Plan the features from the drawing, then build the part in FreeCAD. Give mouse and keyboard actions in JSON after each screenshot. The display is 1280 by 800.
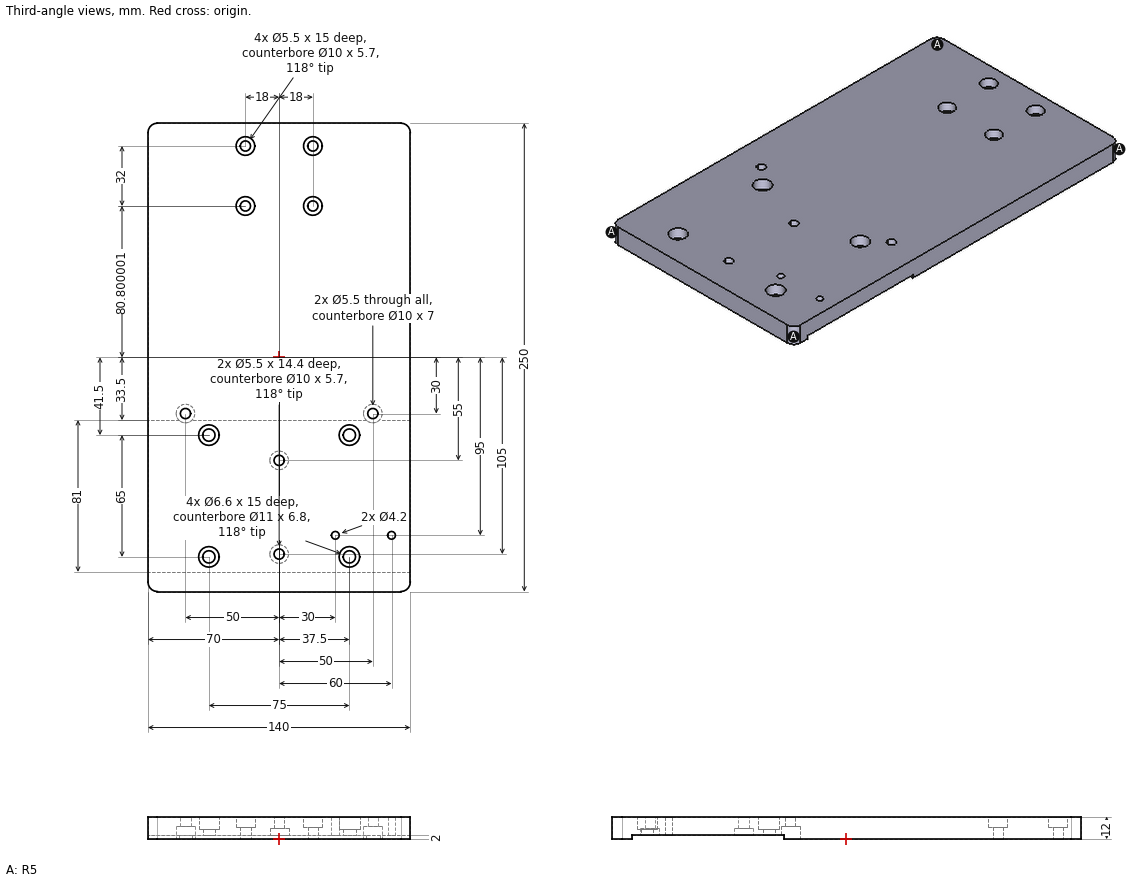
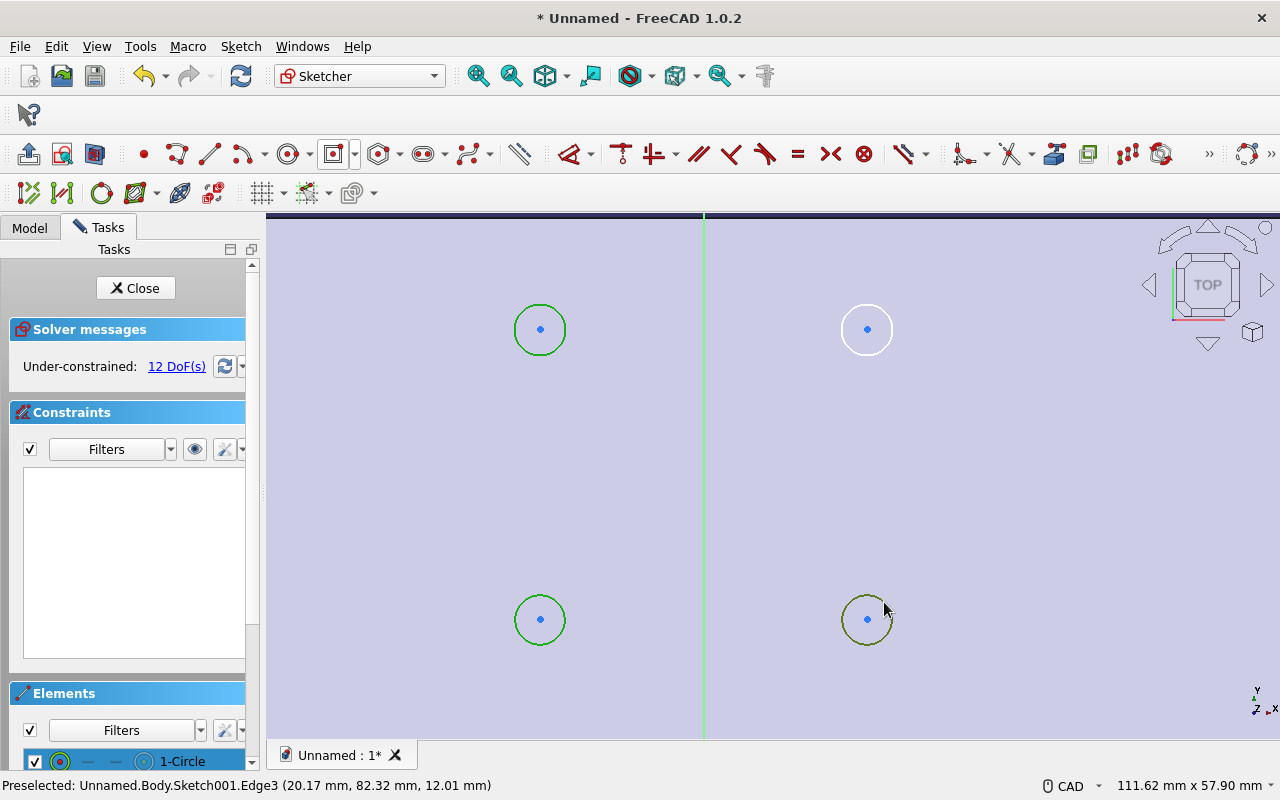
{"action": "left_click", "coordinate": [885, 312]}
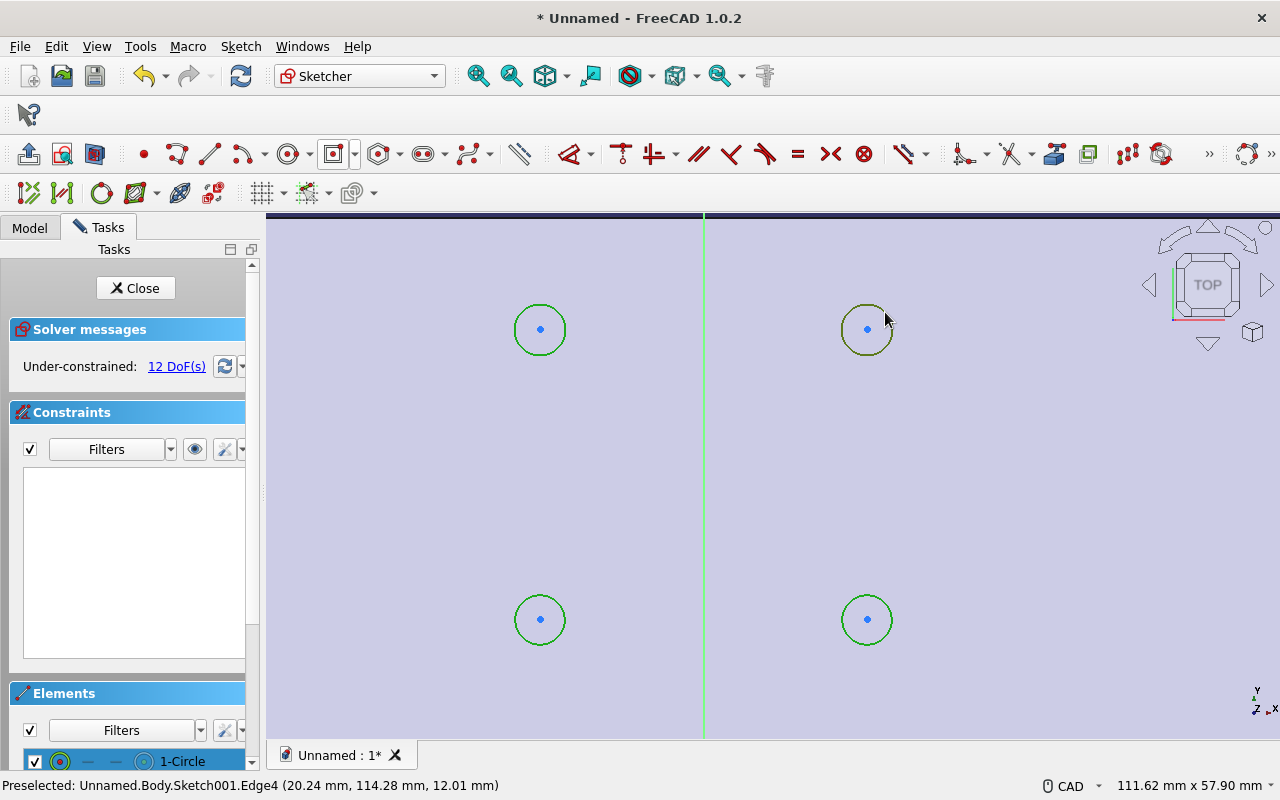
{"action": "left_click", "coordinate": [798, 154]}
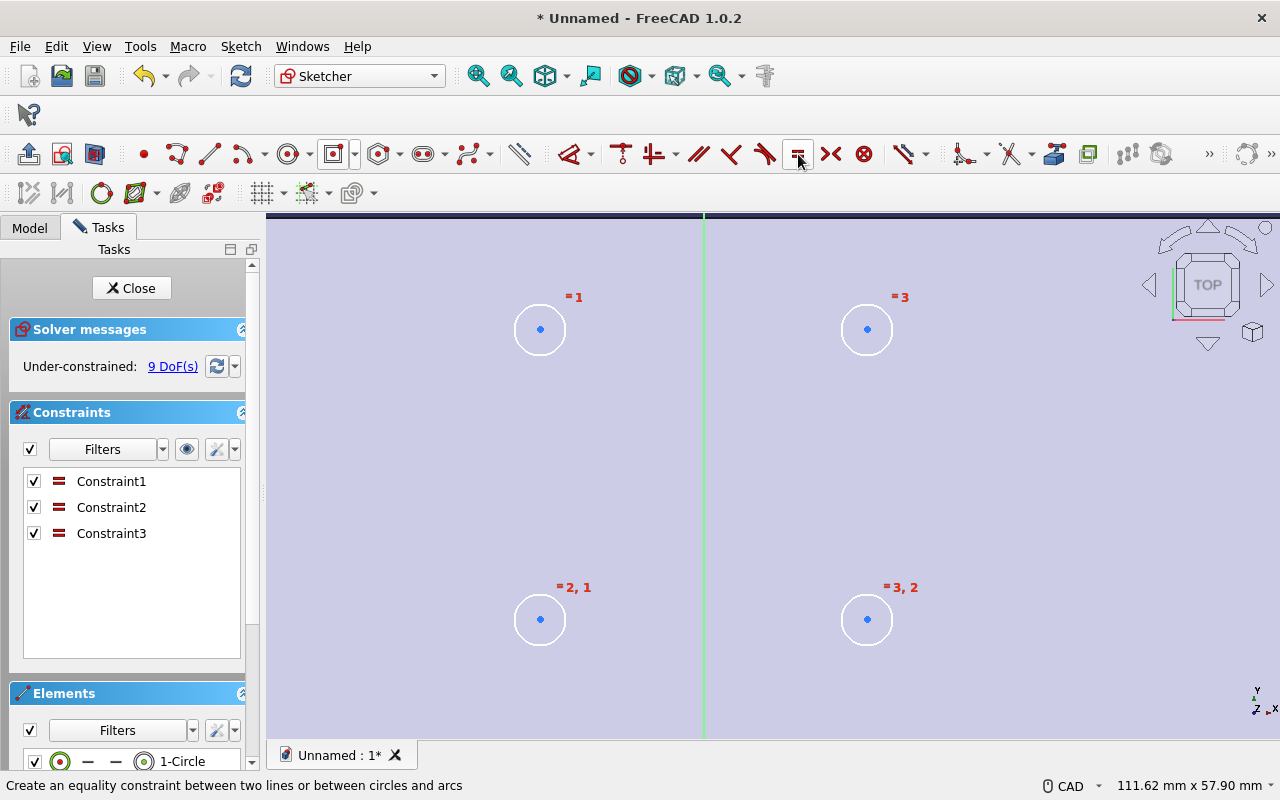
{"action": "left_click", "coordinate": [540, 330]}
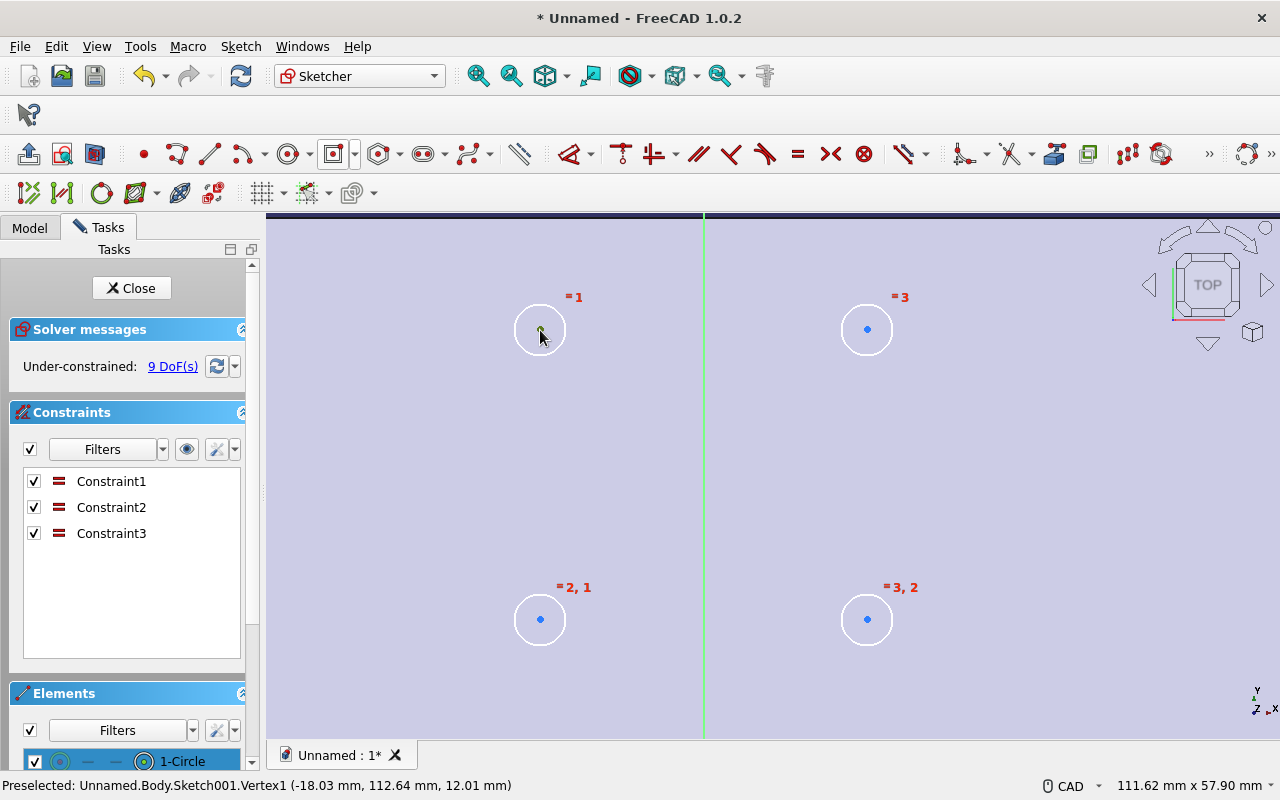
{"action": "left_click", "coordinate": [540, 620]}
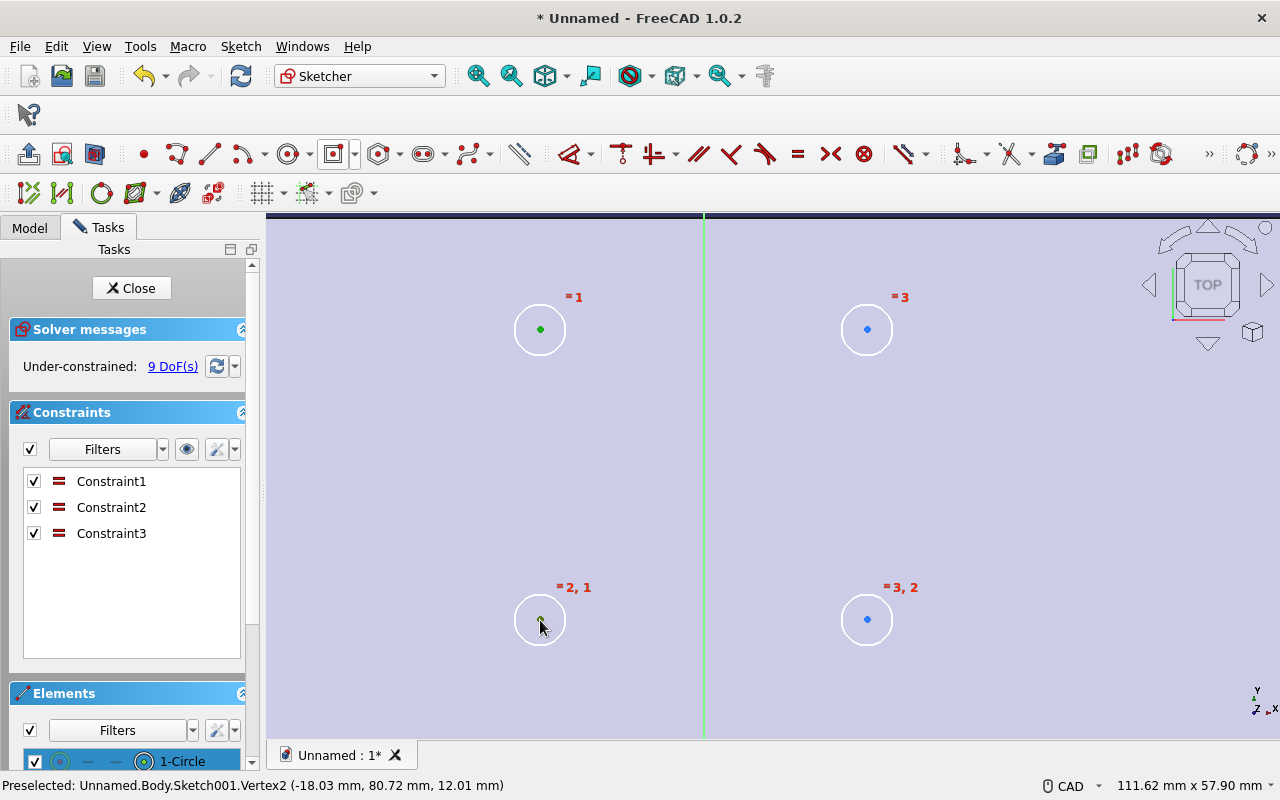
{"action": "key", "text": "v"}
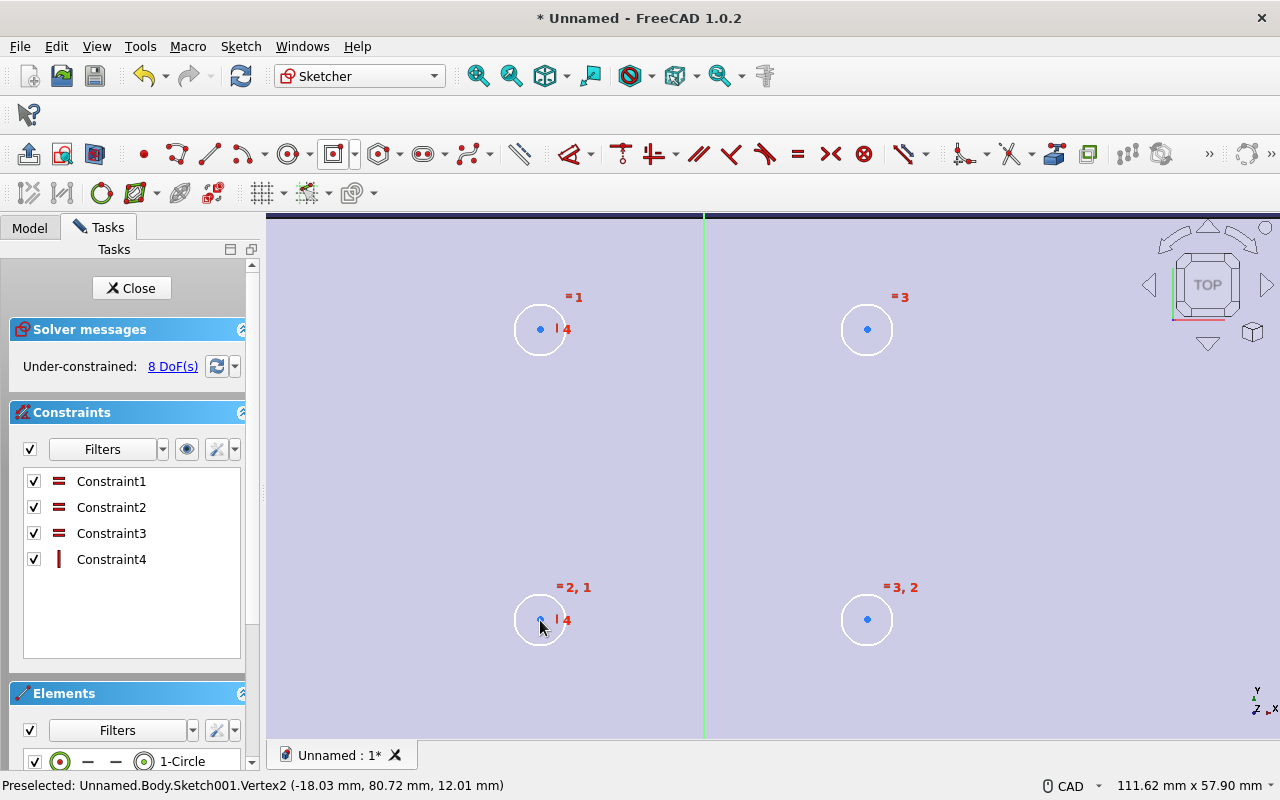
{"action": "left_click", "coordinate": [540, 620]}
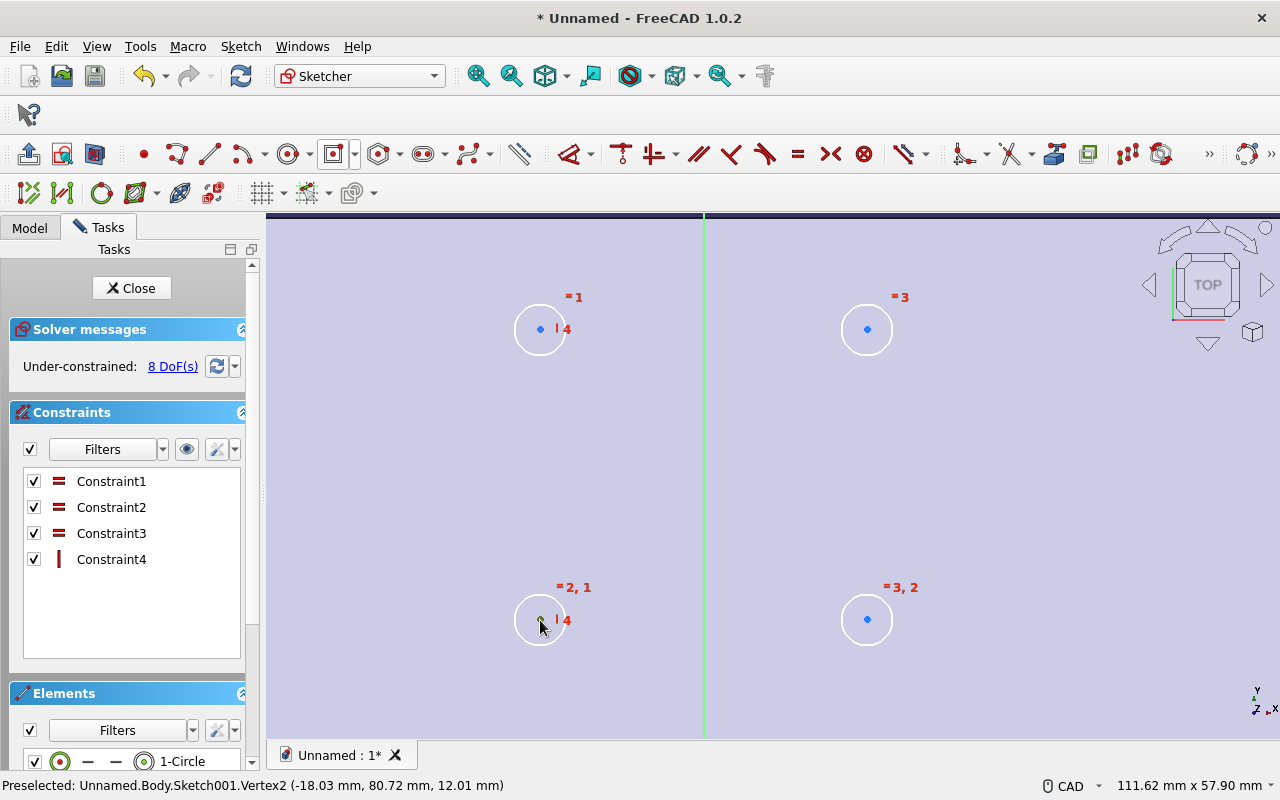
{"action": "left_click", "coordinate": [867, 620]}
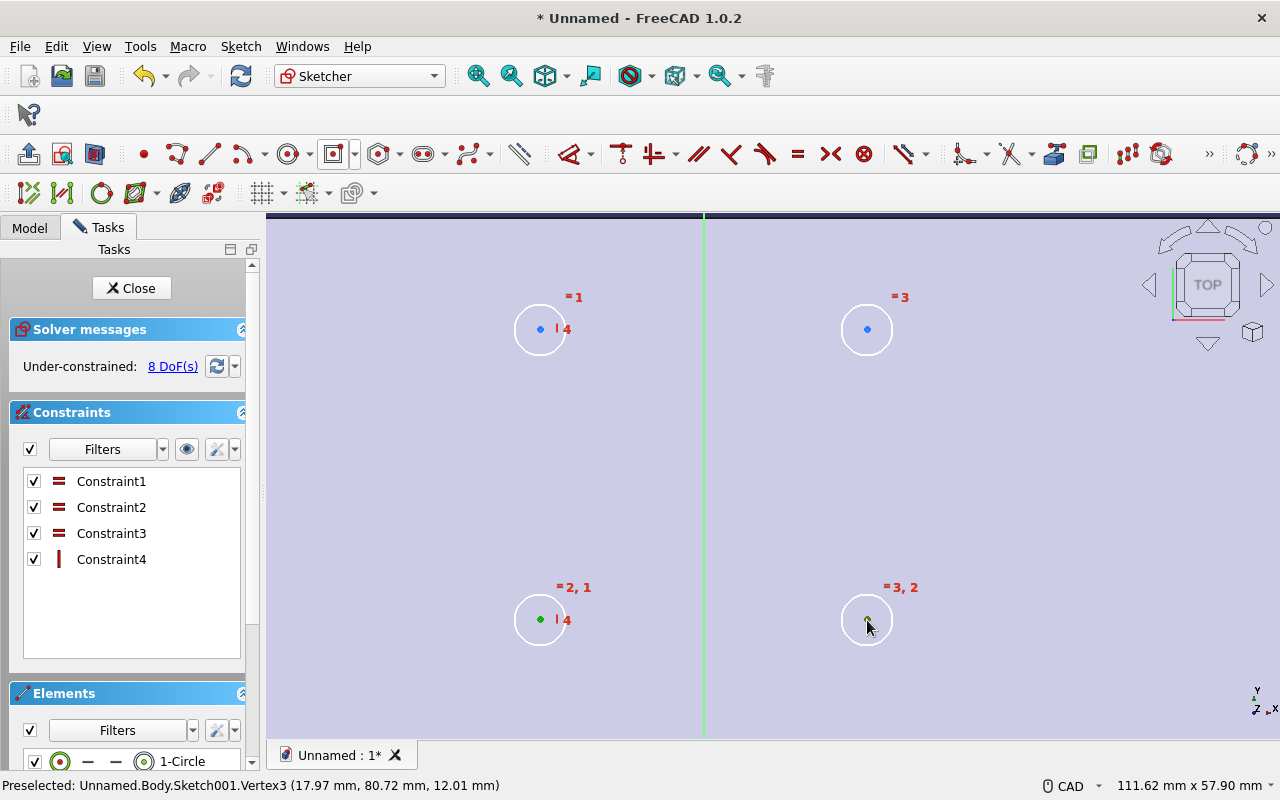
{"action": "left_click", "coordinate": [676, 154]}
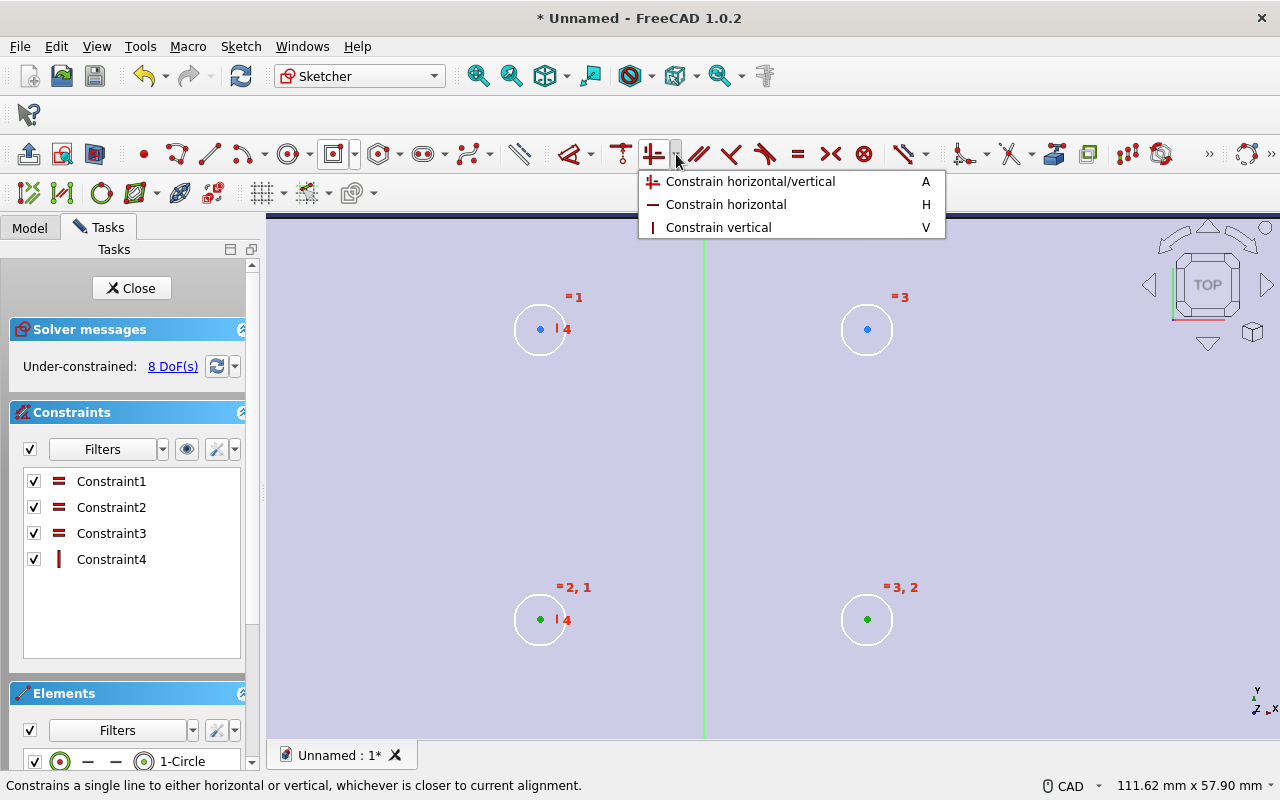
{"action": "left_click", "coordinate": [792, 204]}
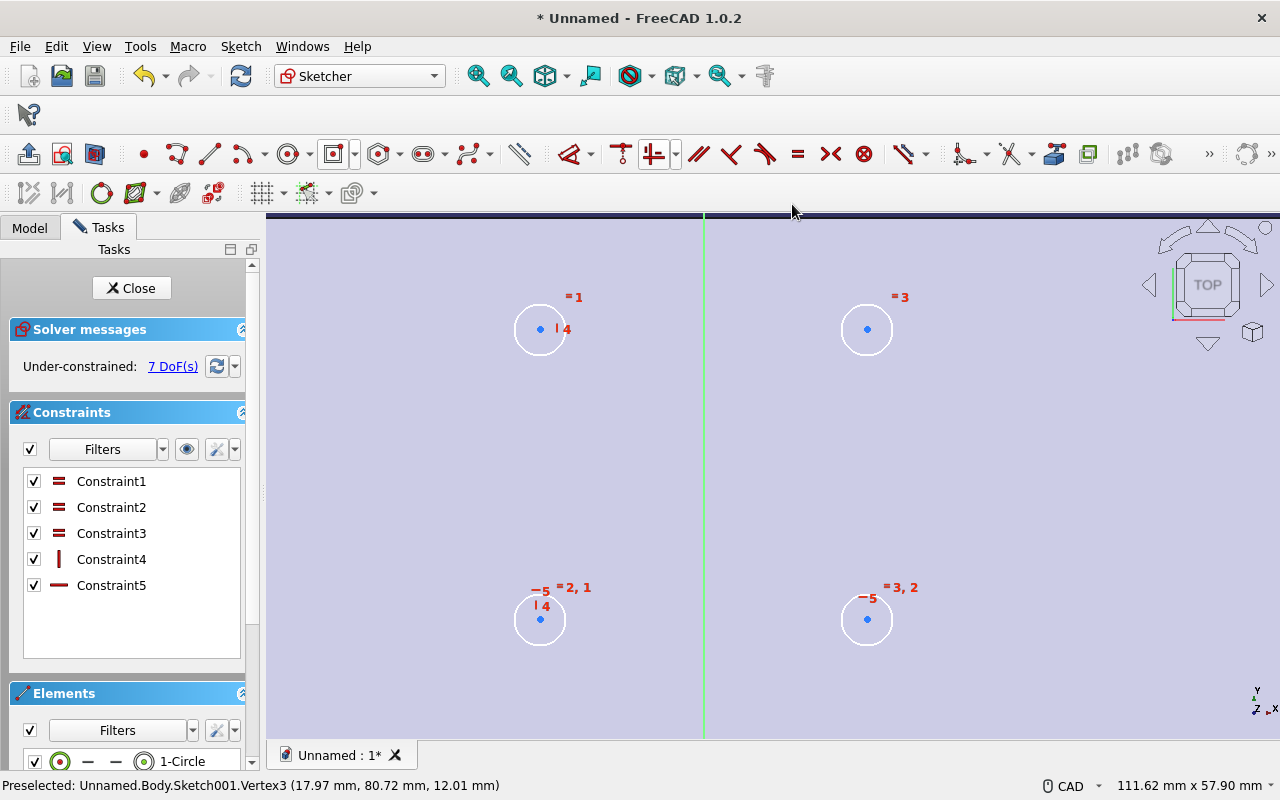
{"action": "left_click", "coordinate": [867, 620]}